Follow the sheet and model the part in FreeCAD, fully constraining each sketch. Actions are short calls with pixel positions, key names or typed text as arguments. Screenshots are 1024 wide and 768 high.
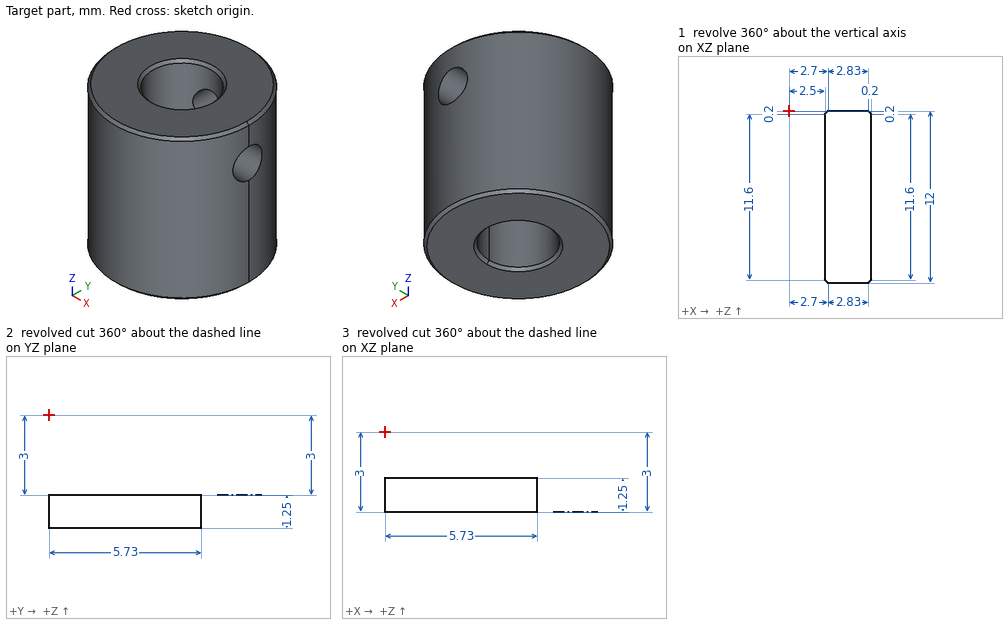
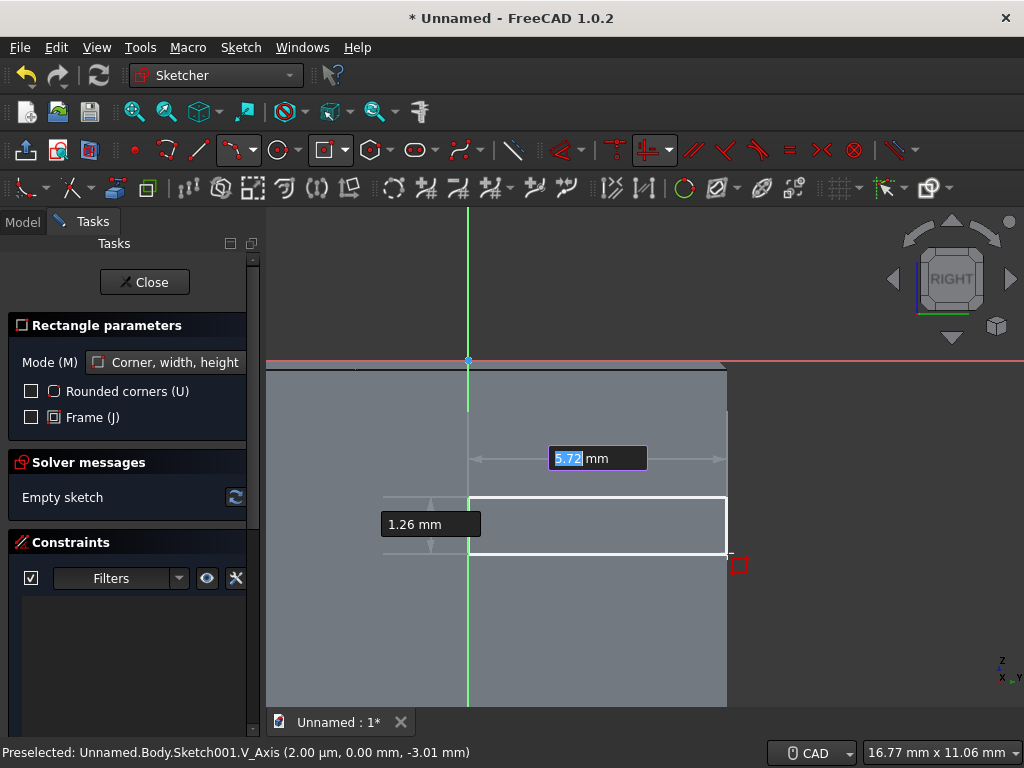
text(5.73)
key(Tab)
text(1.25)
key(Return)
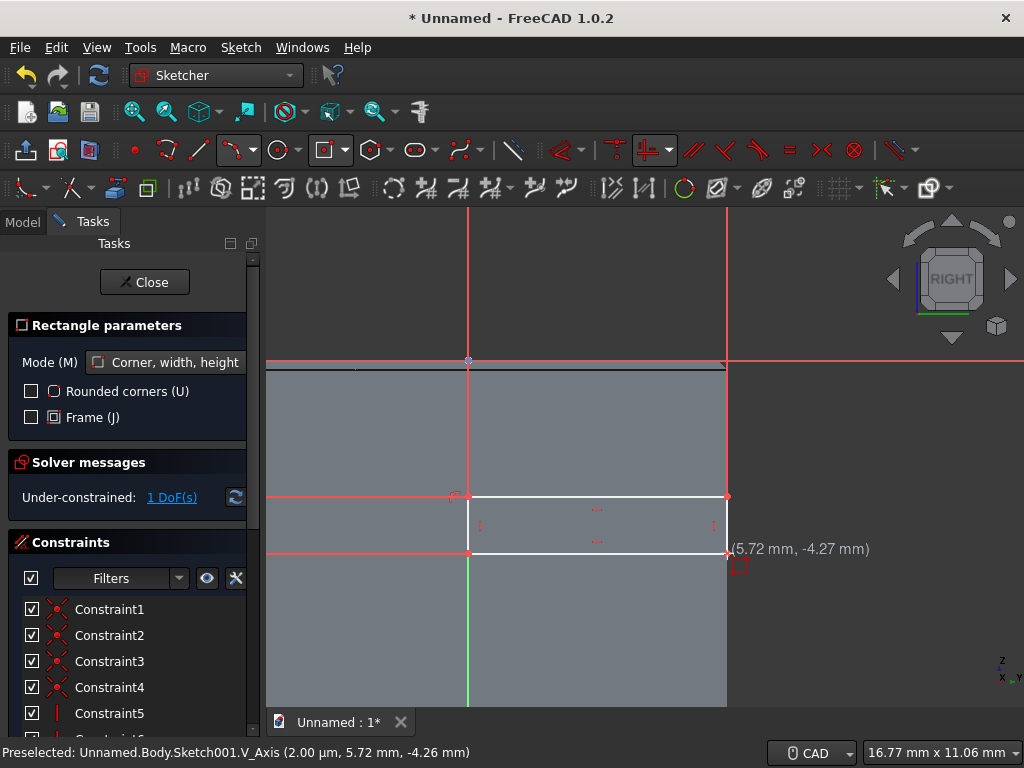
key(g)
key(l)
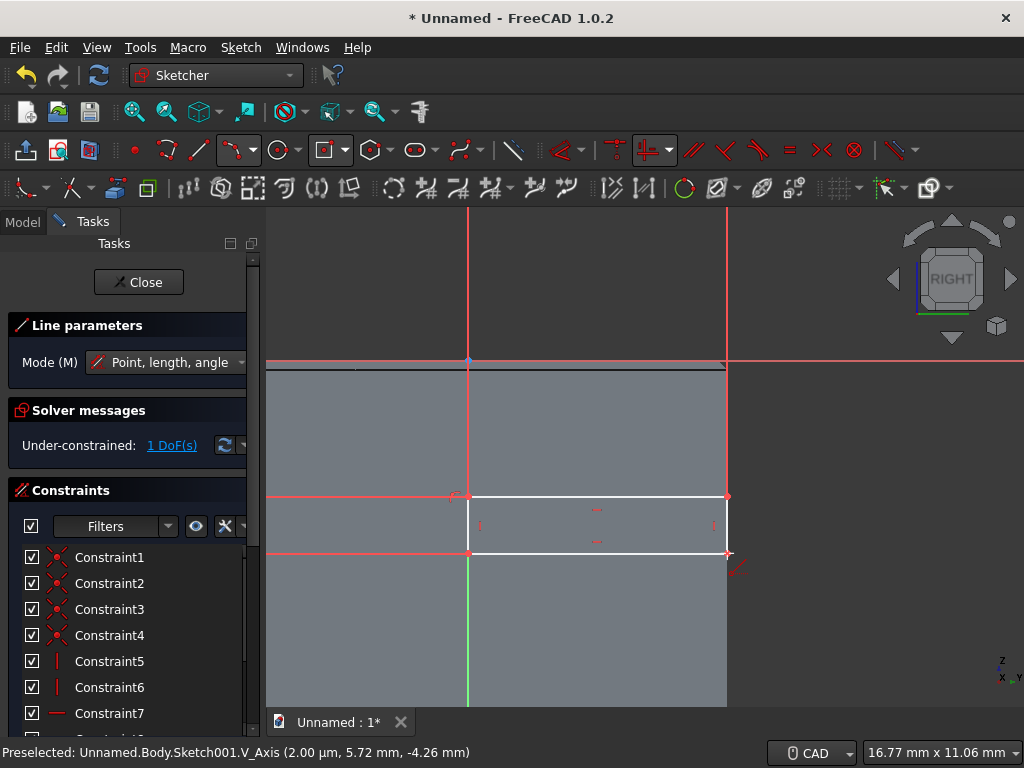
click(753, 496)
click(831, 496)
key(Escape)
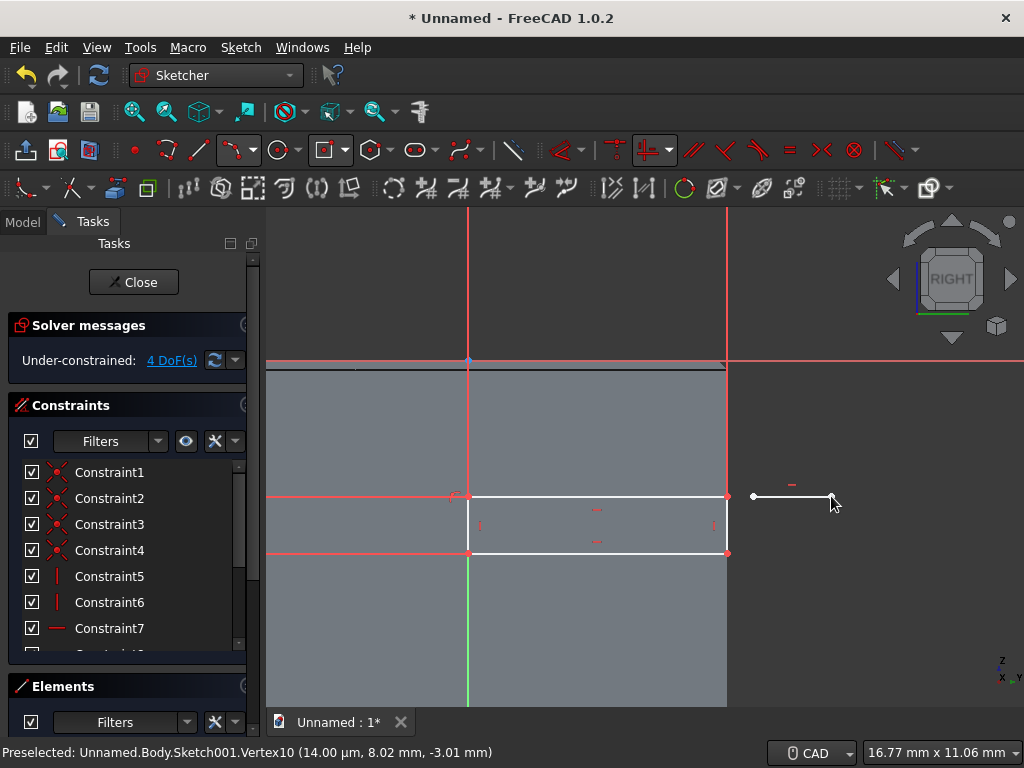
click(776, 497)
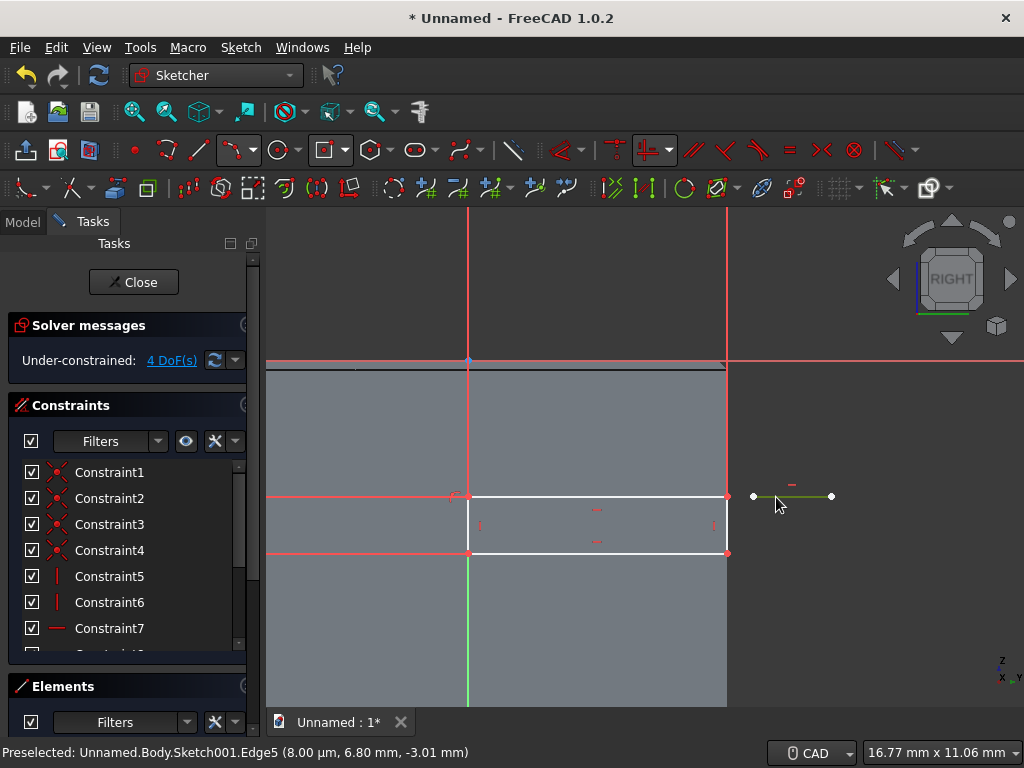
click(514, 150)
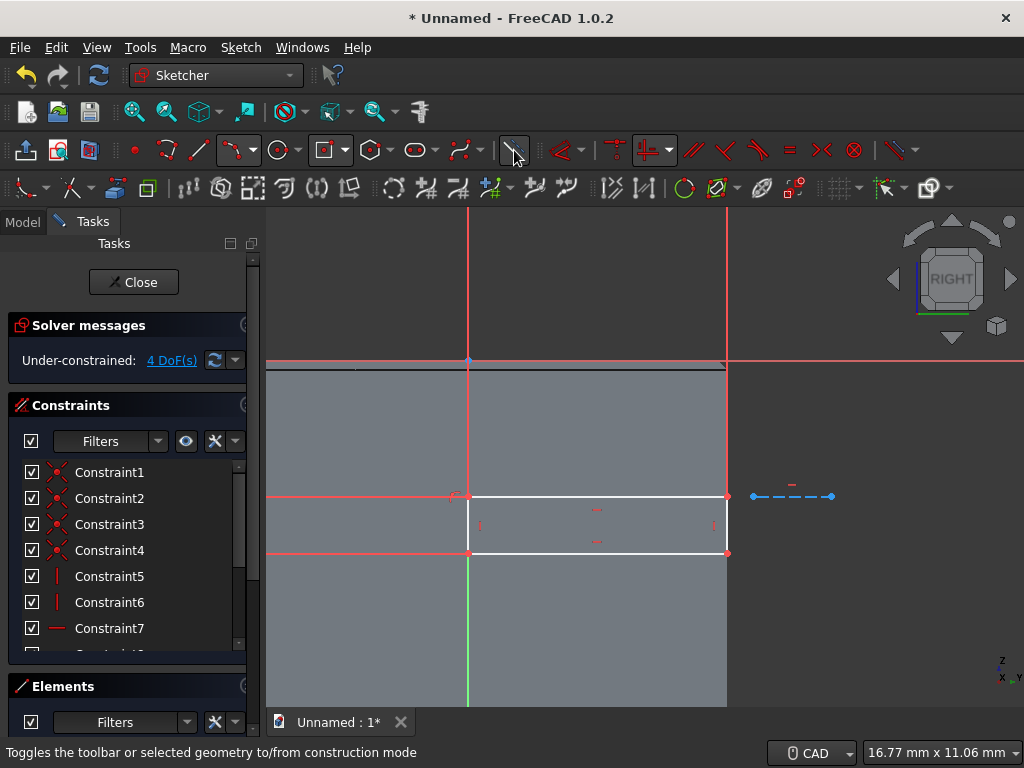
click(560, 150)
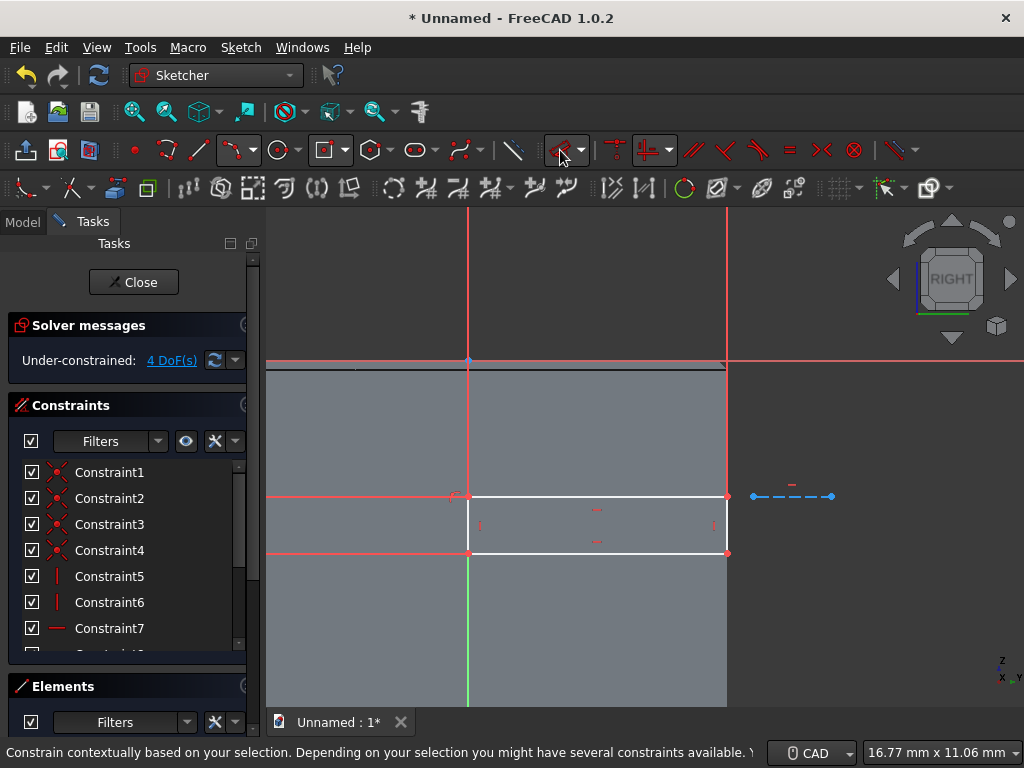
click(468, 497)
click(434, 429)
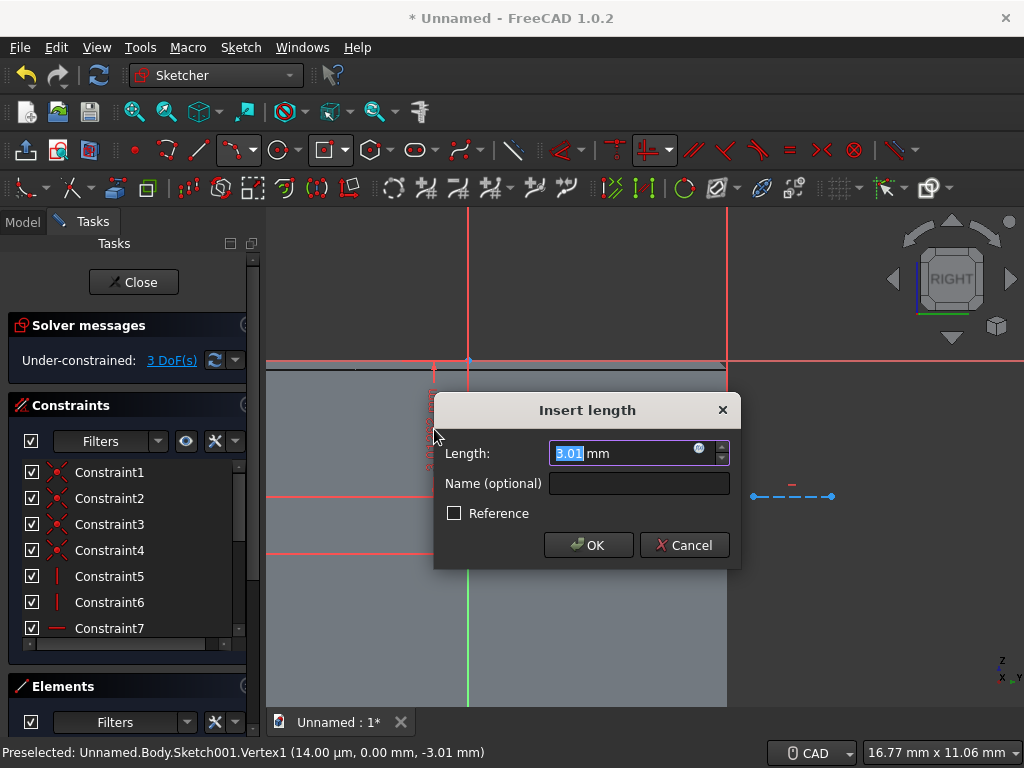
text(3)
key(Return)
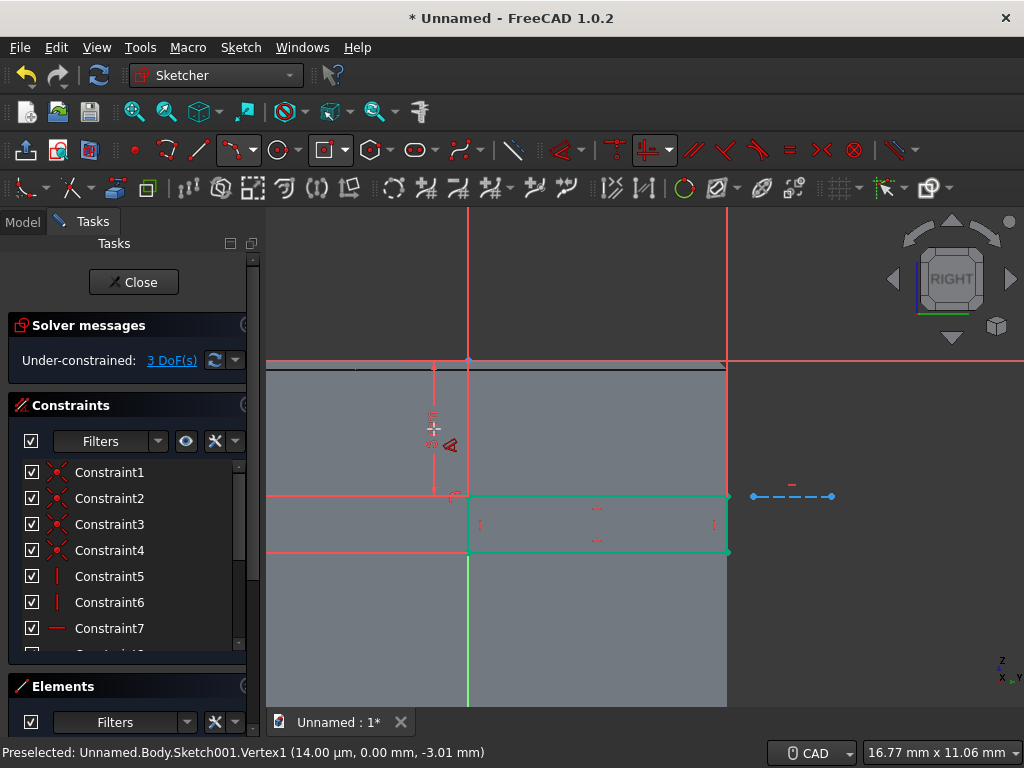
click(753, 497)
click(434, 398)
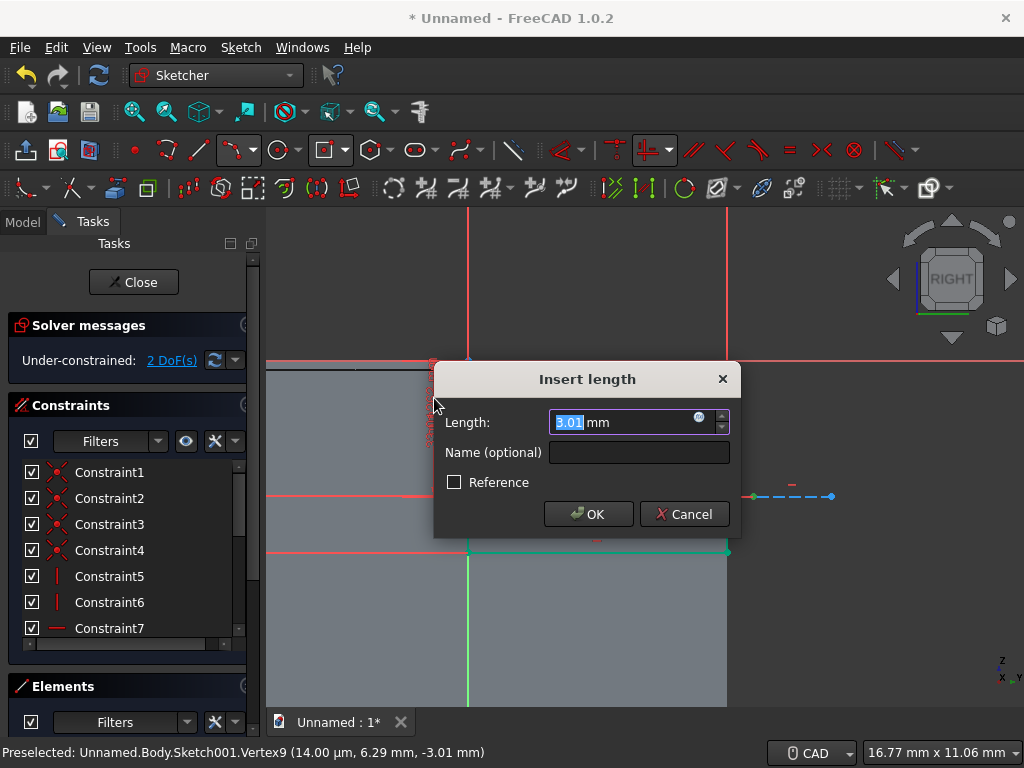
text(3)
key(Return)
key(Escape)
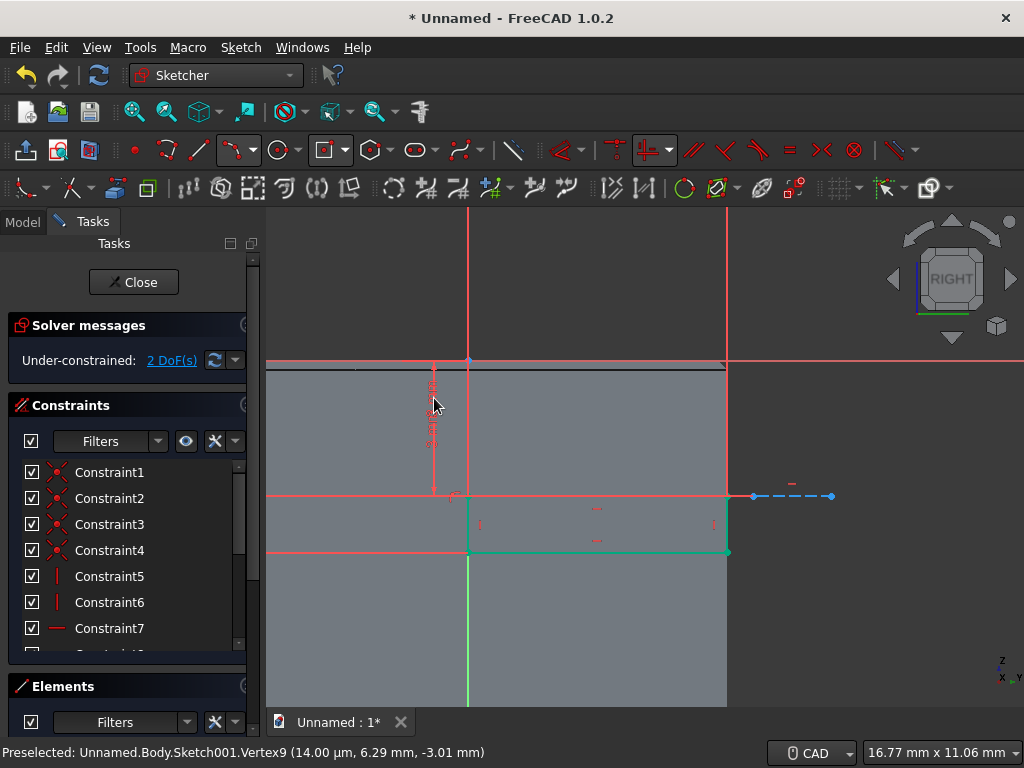
click(134, 282)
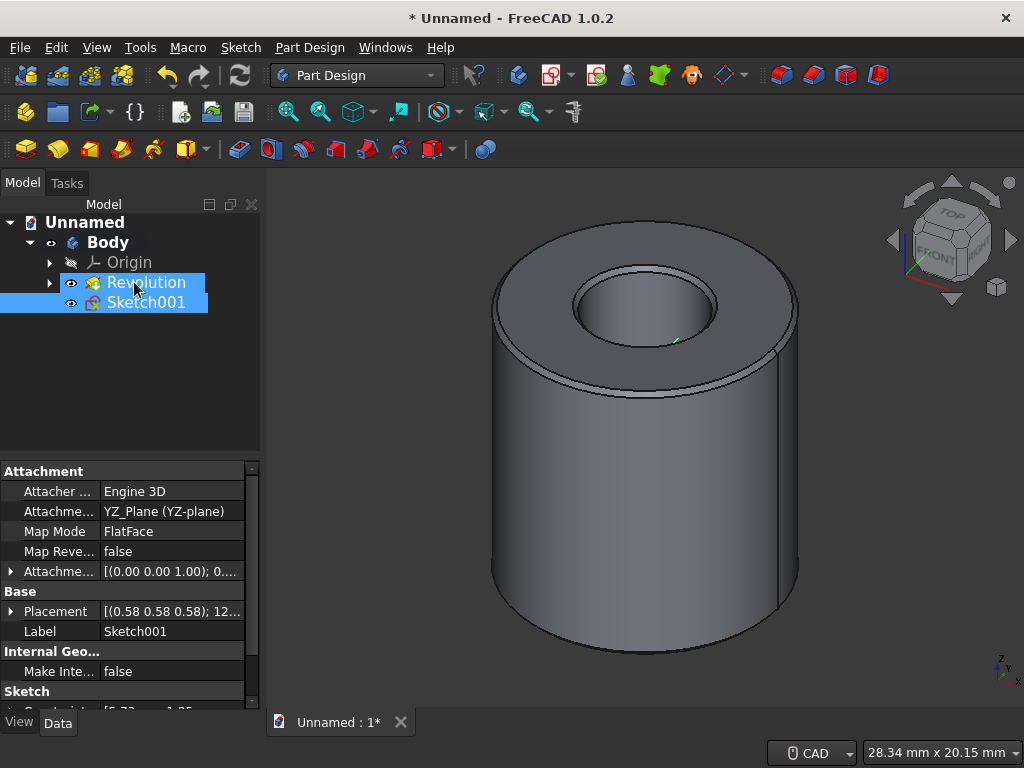
click(304, 150)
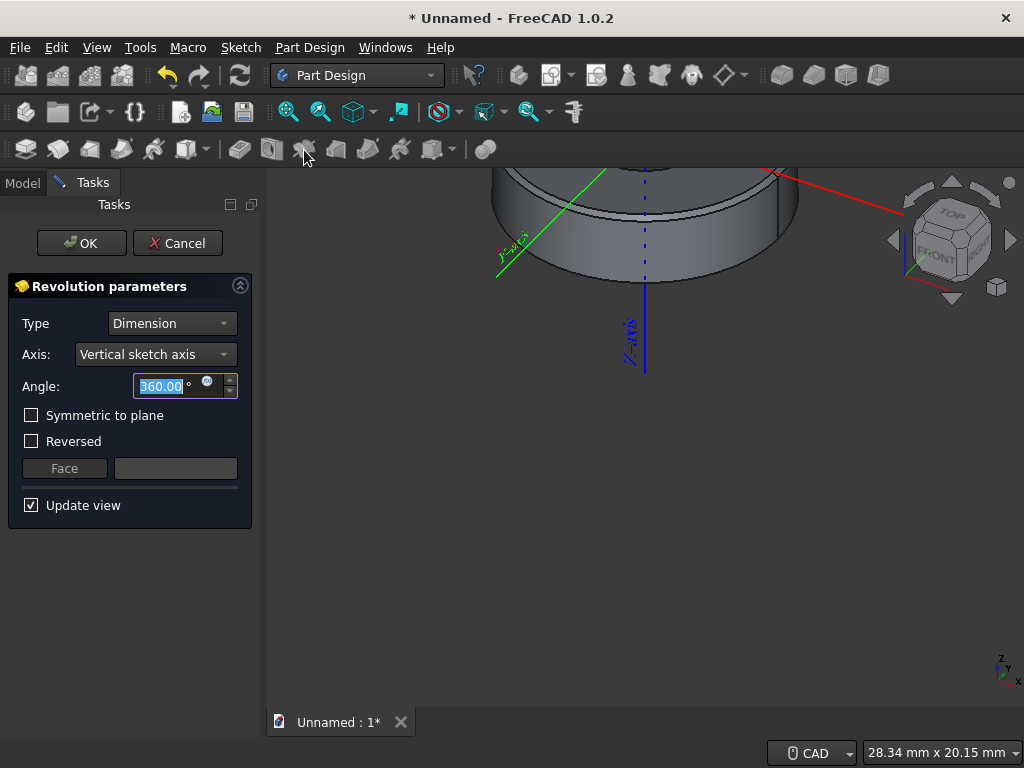
click(156, 354)